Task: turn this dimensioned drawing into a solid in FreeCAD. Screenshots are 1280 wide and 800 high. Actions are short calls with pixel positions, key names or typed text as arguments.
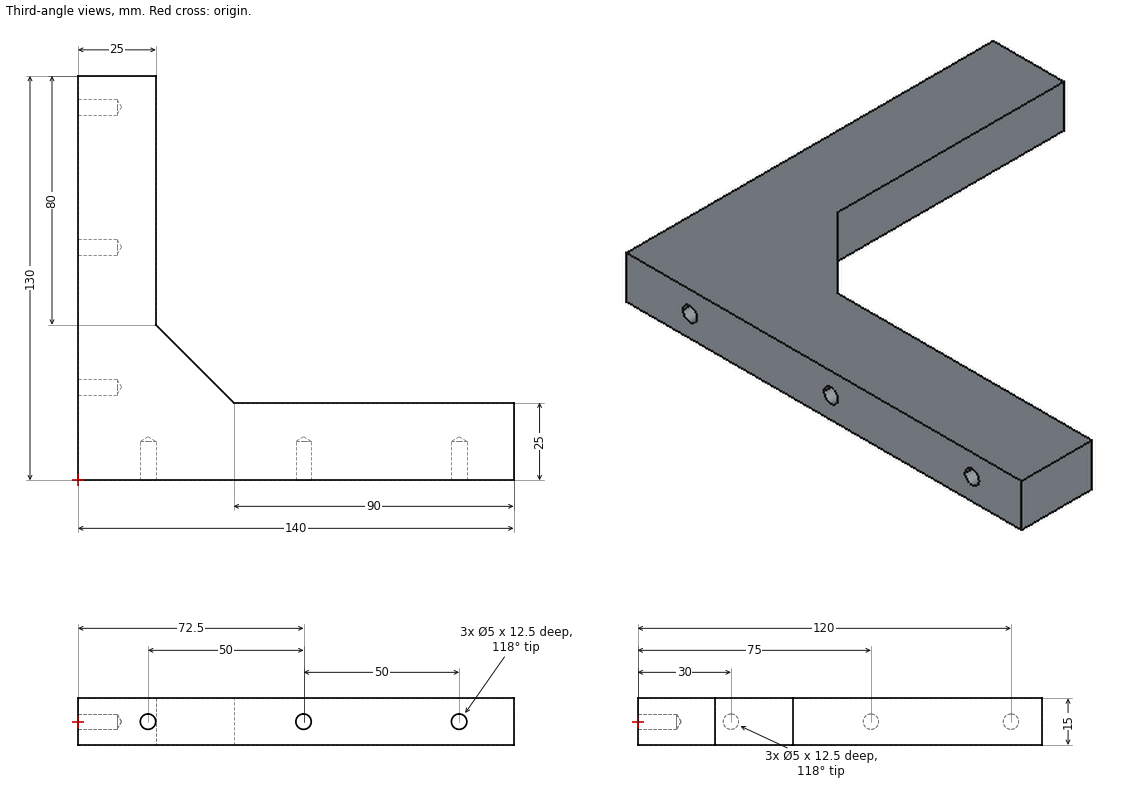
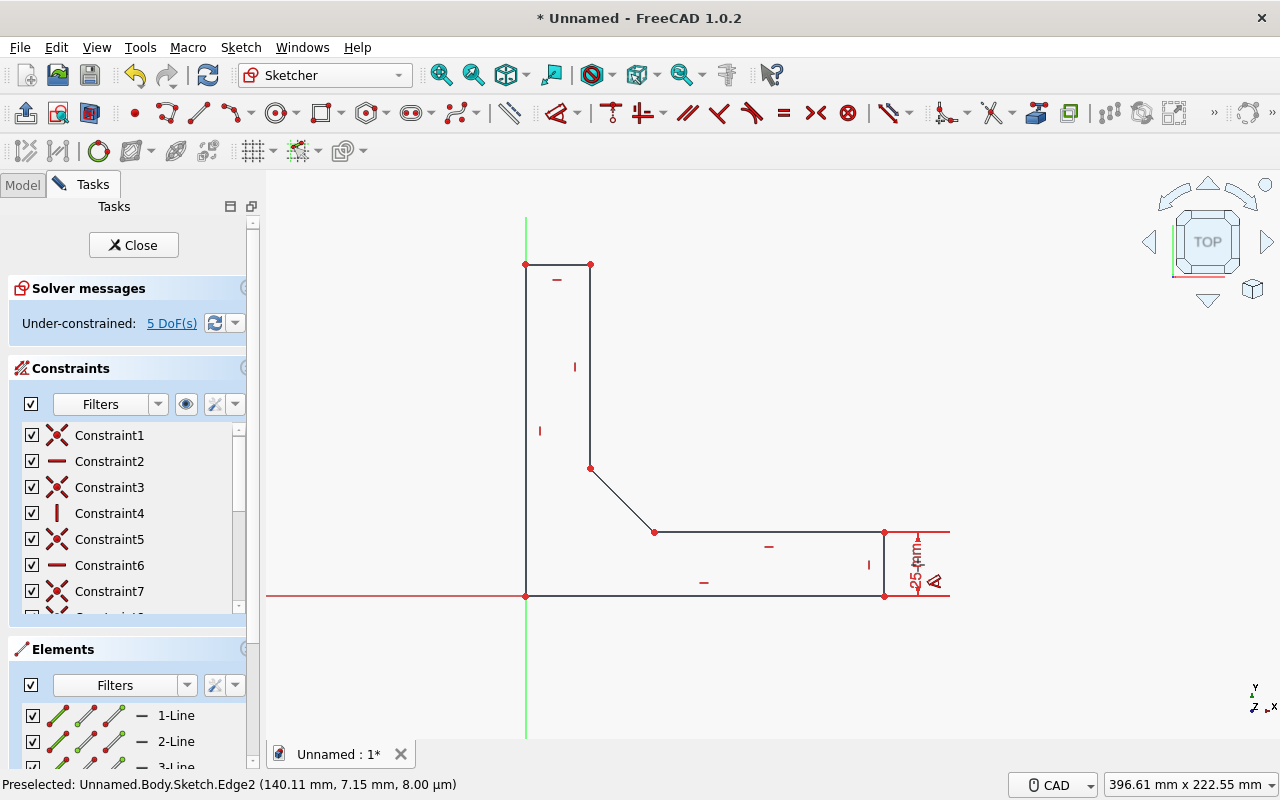
click(815, 532)
click(769, 566)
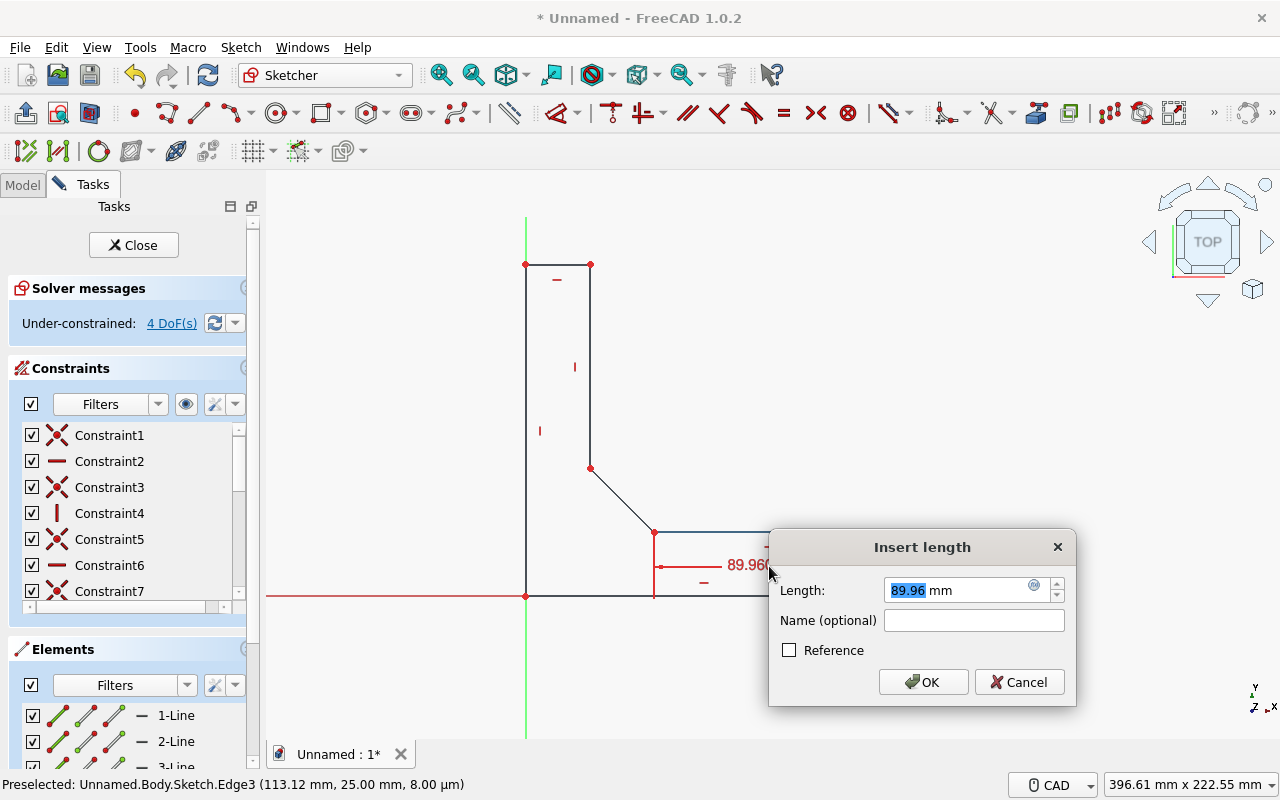
text(90)
key(Return)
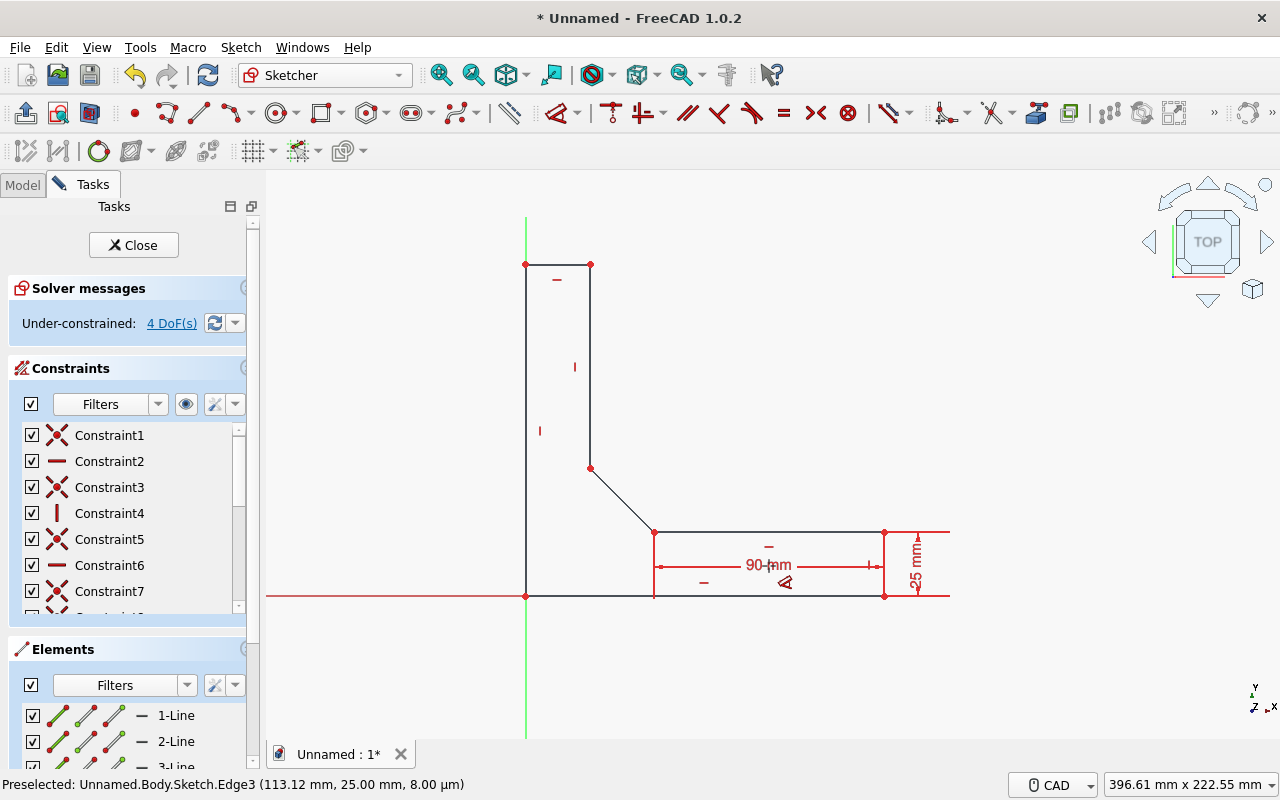
click(590, 408)
click(556, 367)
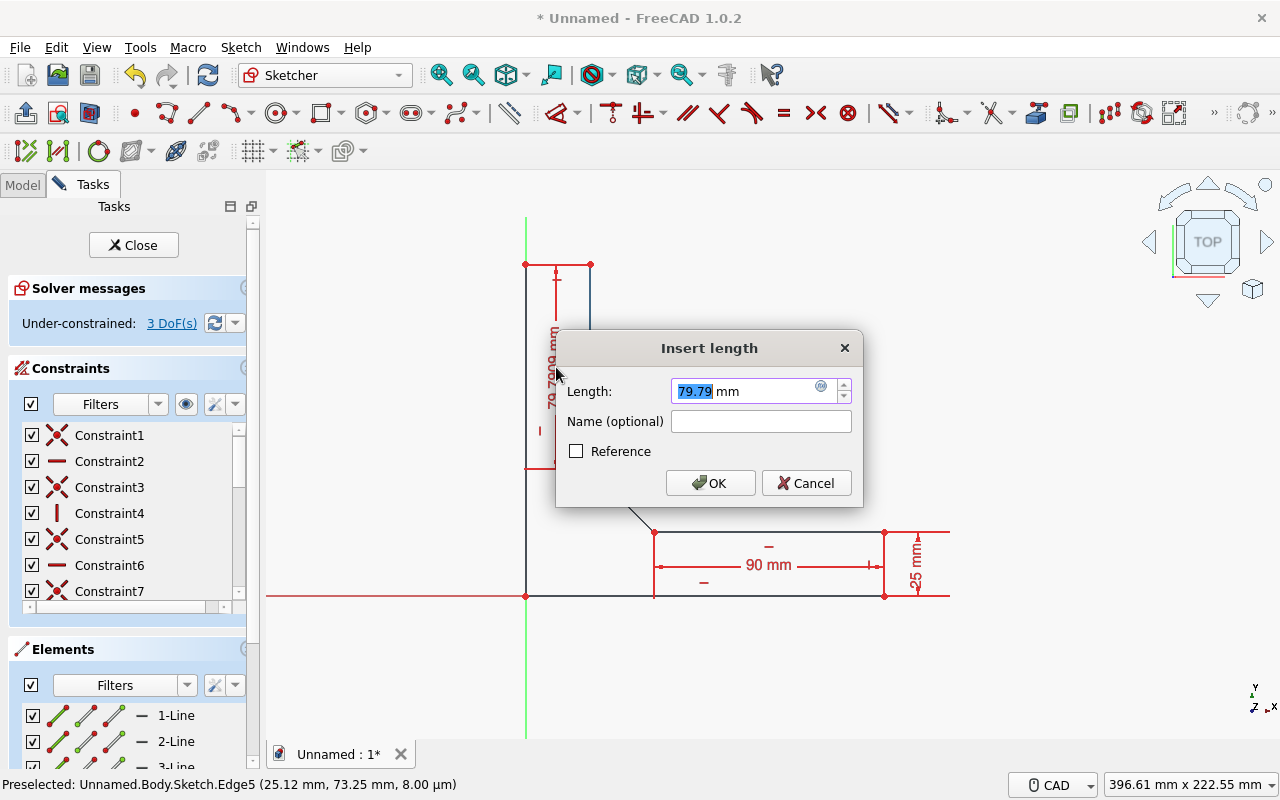
text(80)
key(Return)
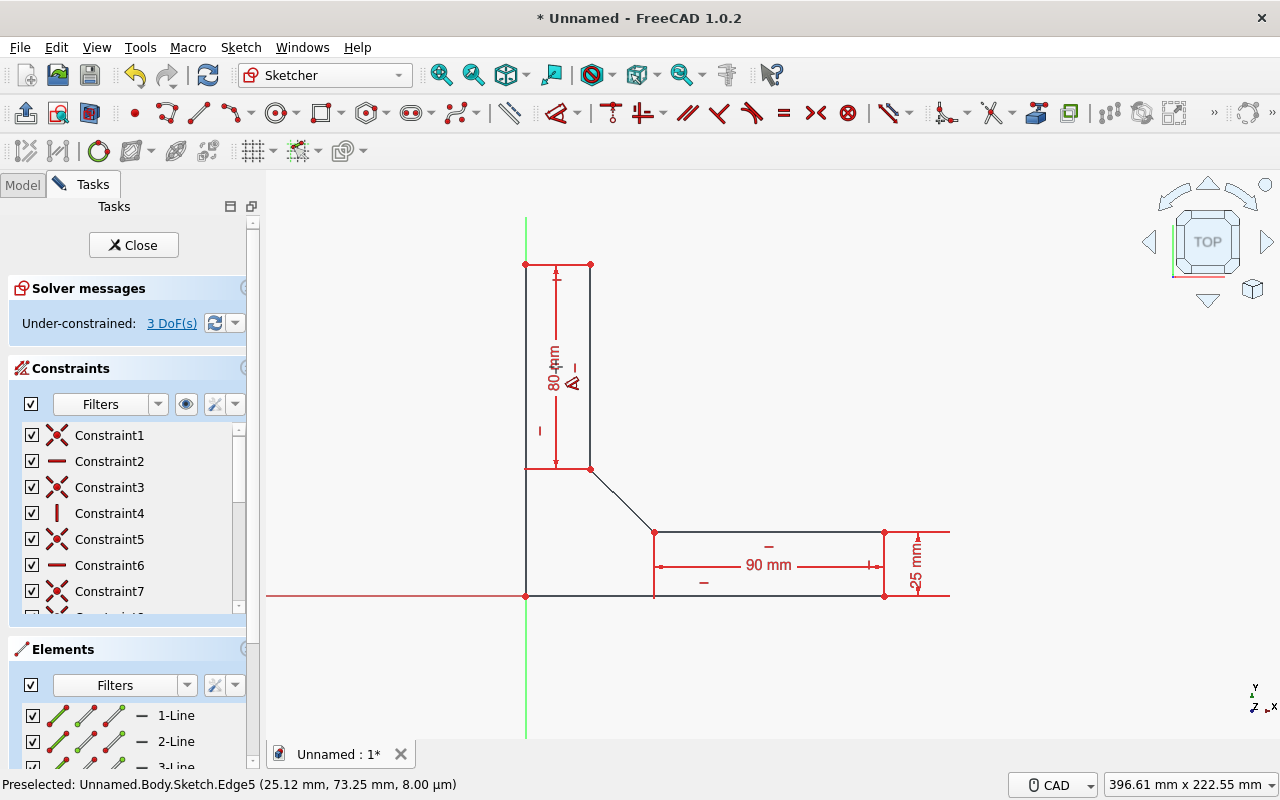
click(571, 265)
click(558, 231)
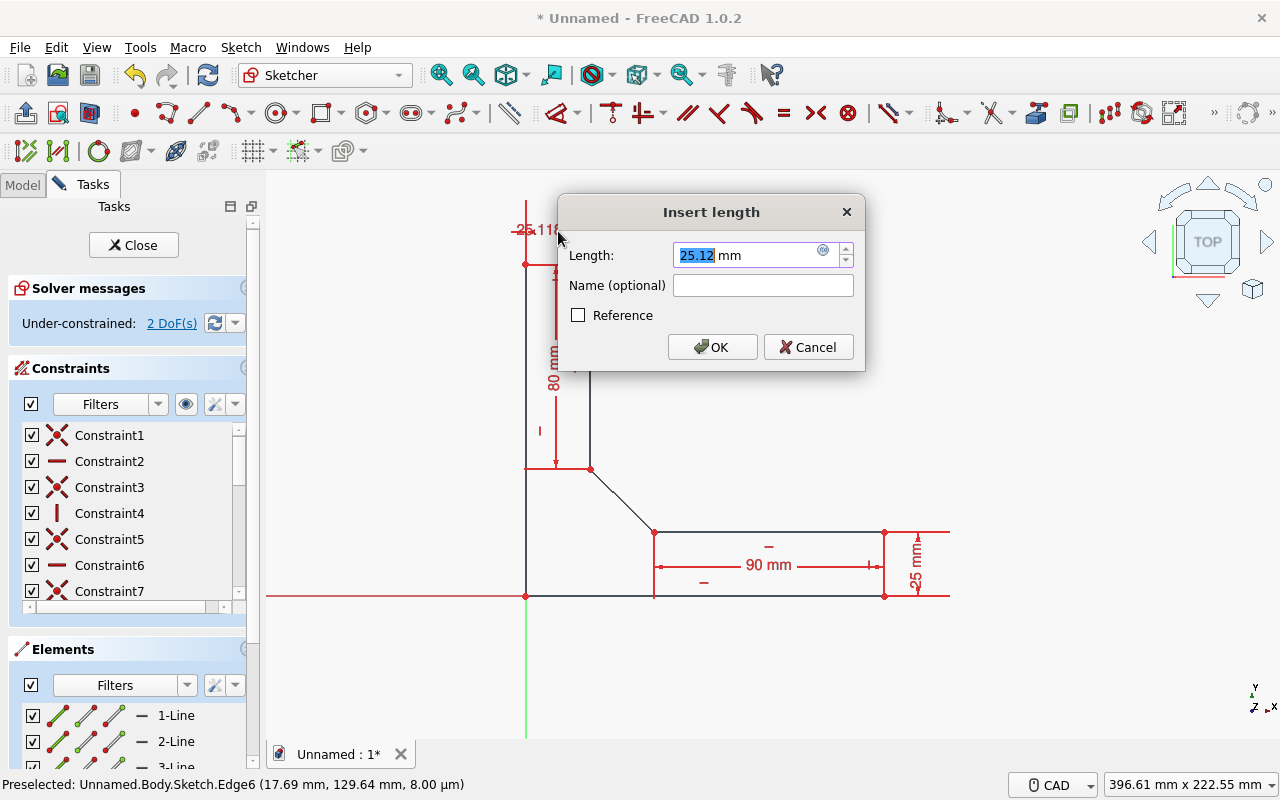
text(25)
key(Return)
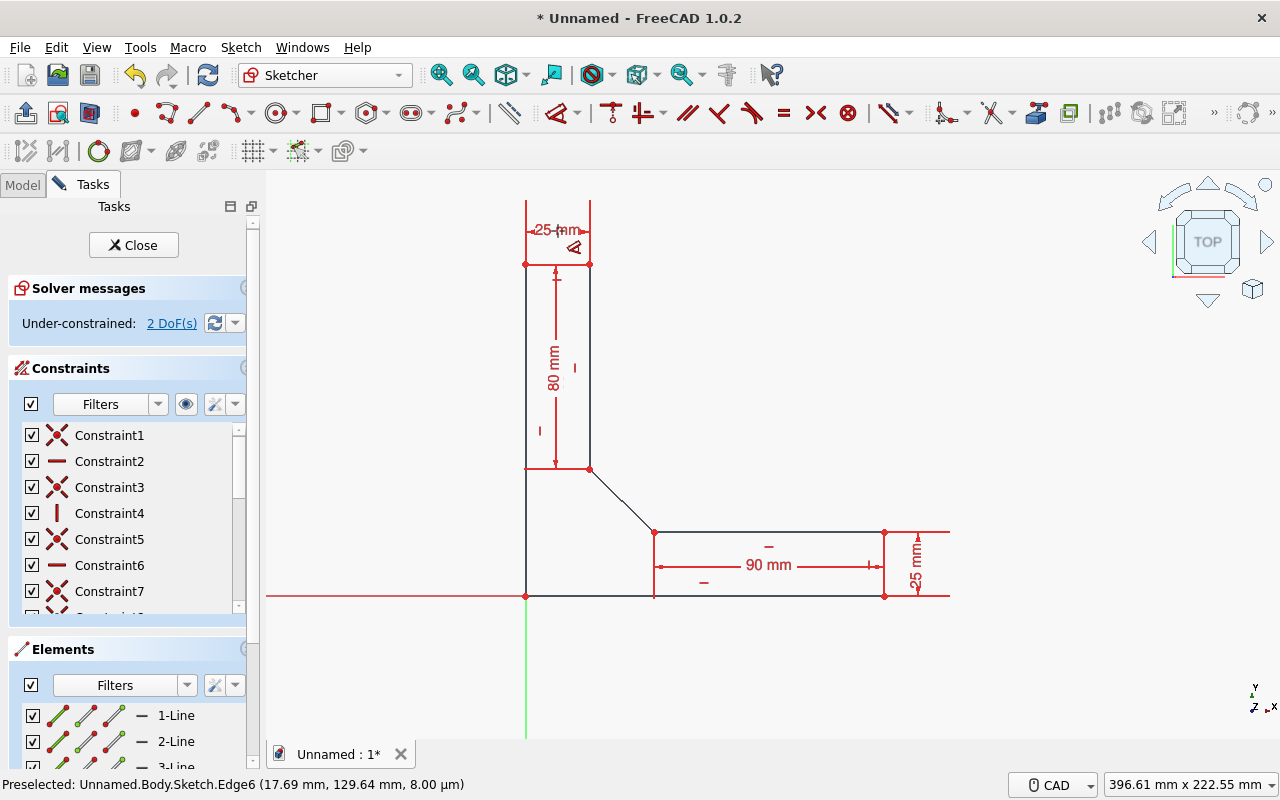
click(633, 596)
click(705, 630)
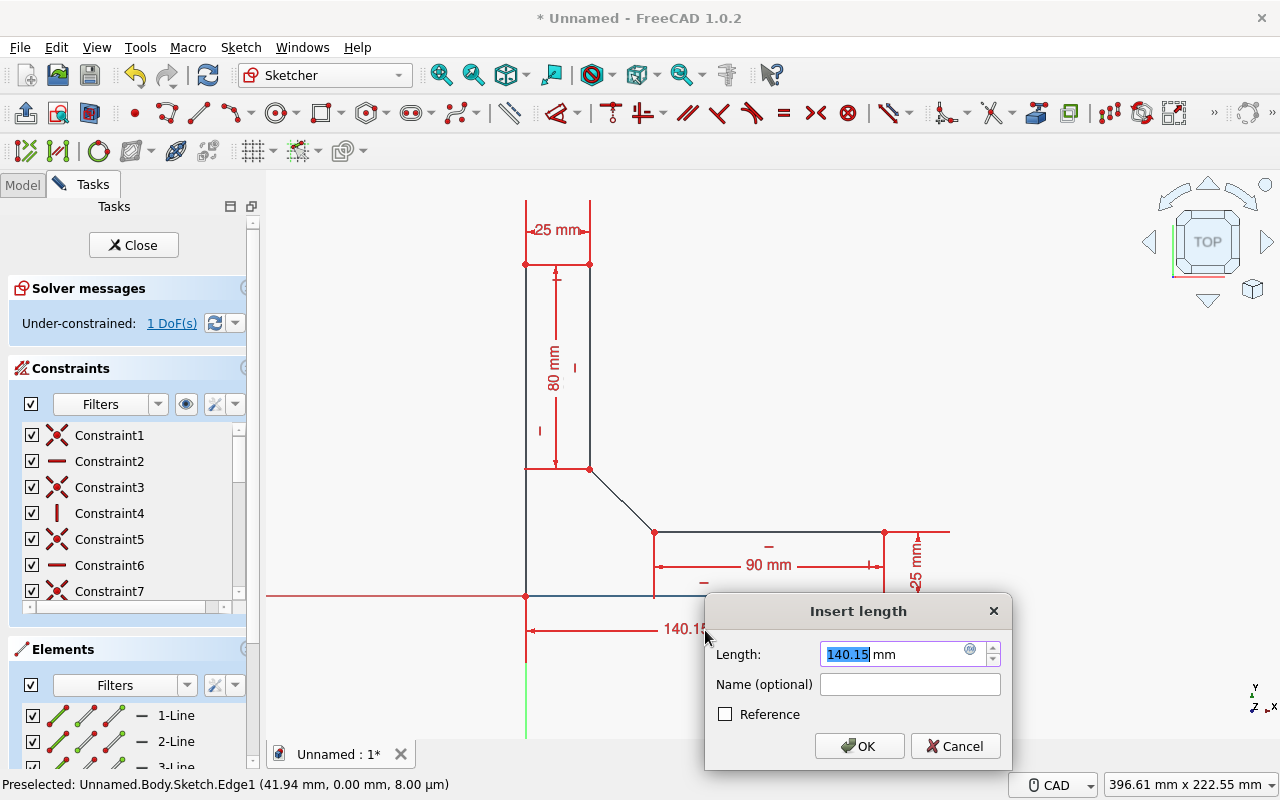
text(140)
key(Return)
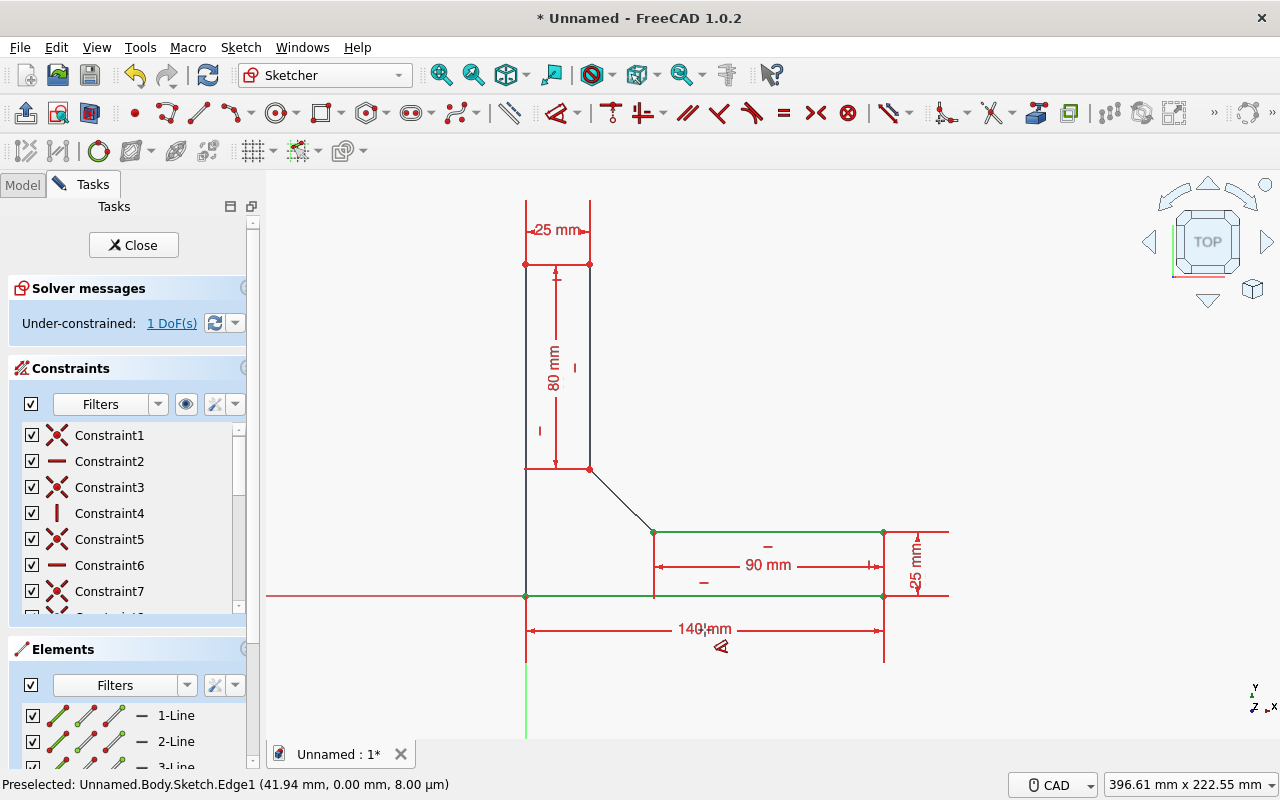
click(526, 364)
click(492, 431)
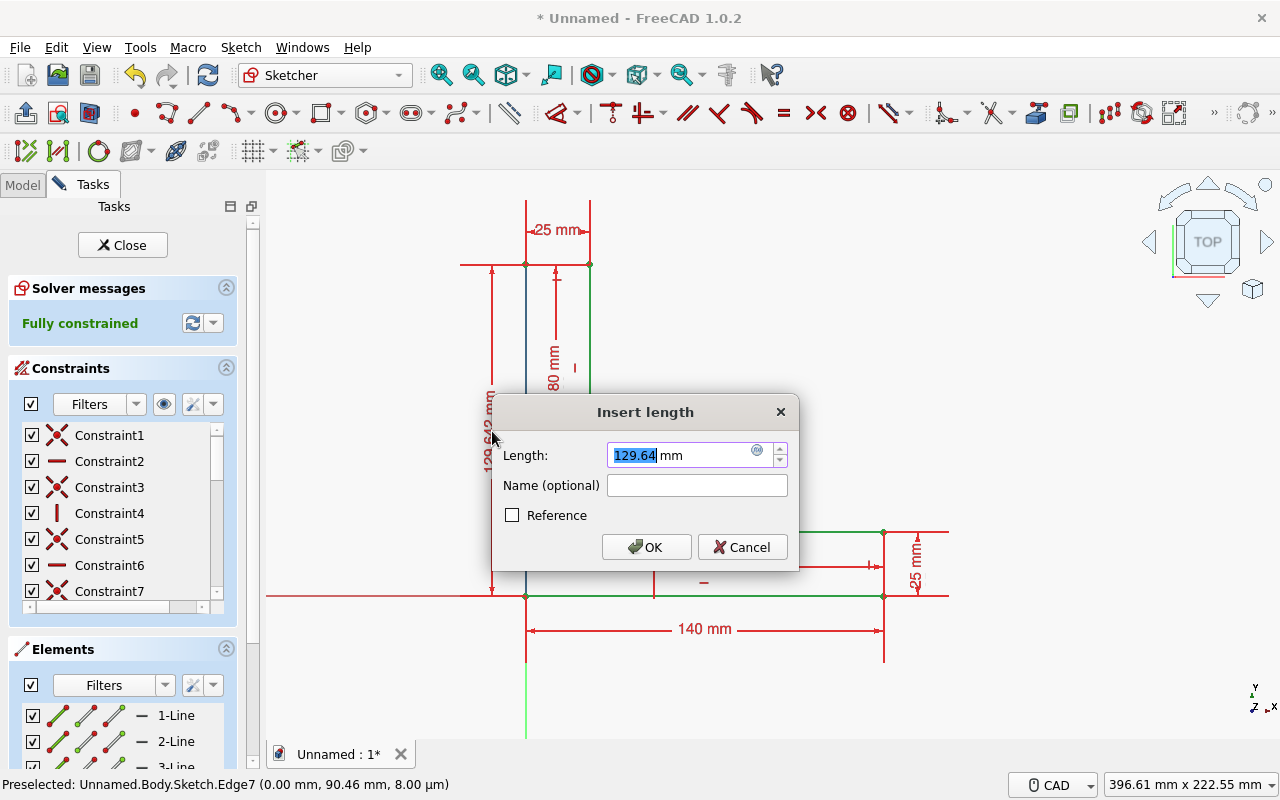
text(130)
key(Return)
key(Escape)